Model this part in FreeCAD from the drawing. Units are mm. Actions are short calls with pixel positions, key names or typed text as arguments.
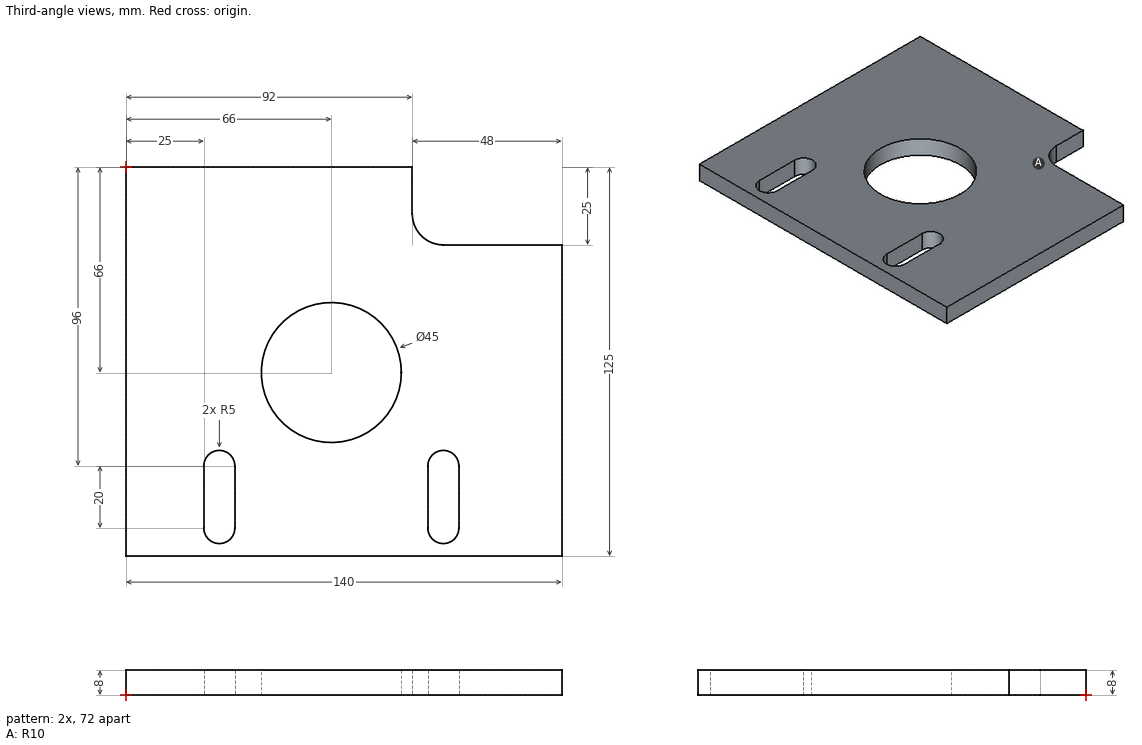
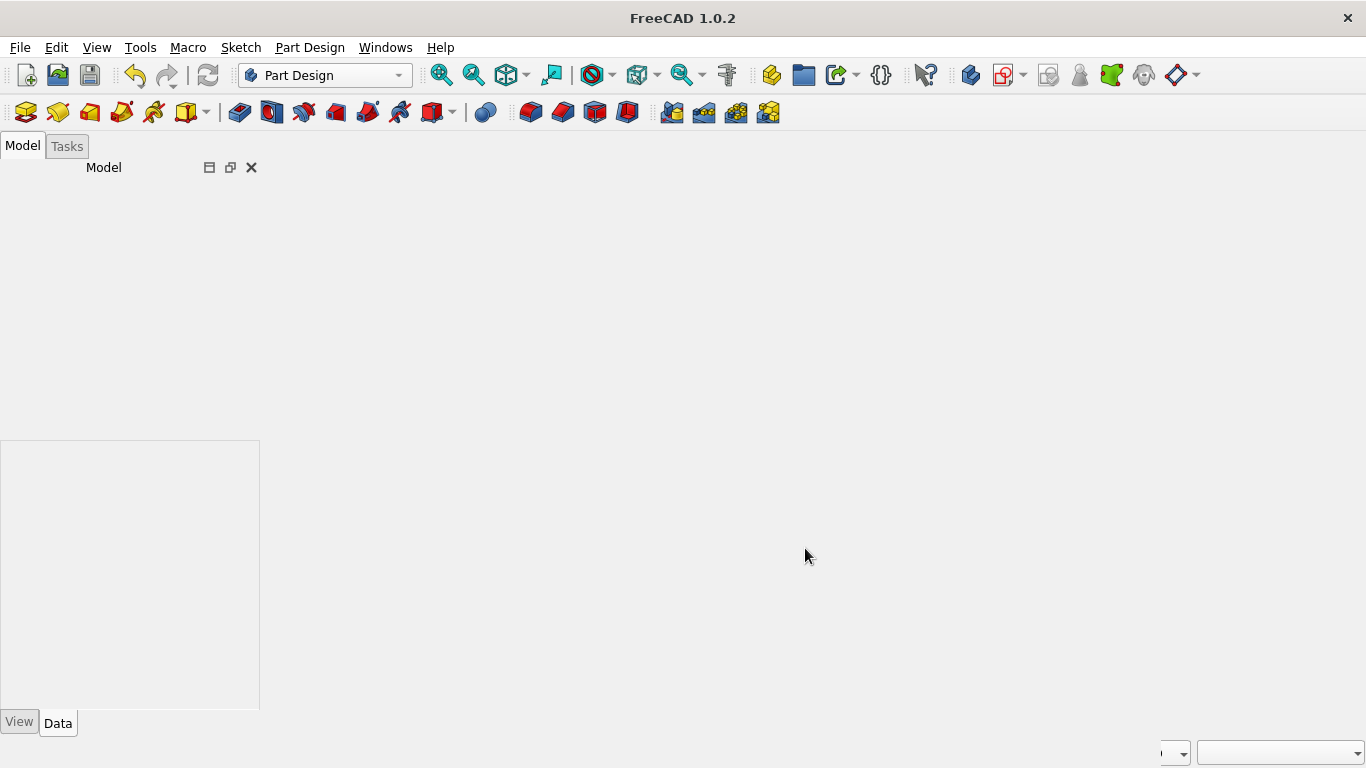
click(26, 76)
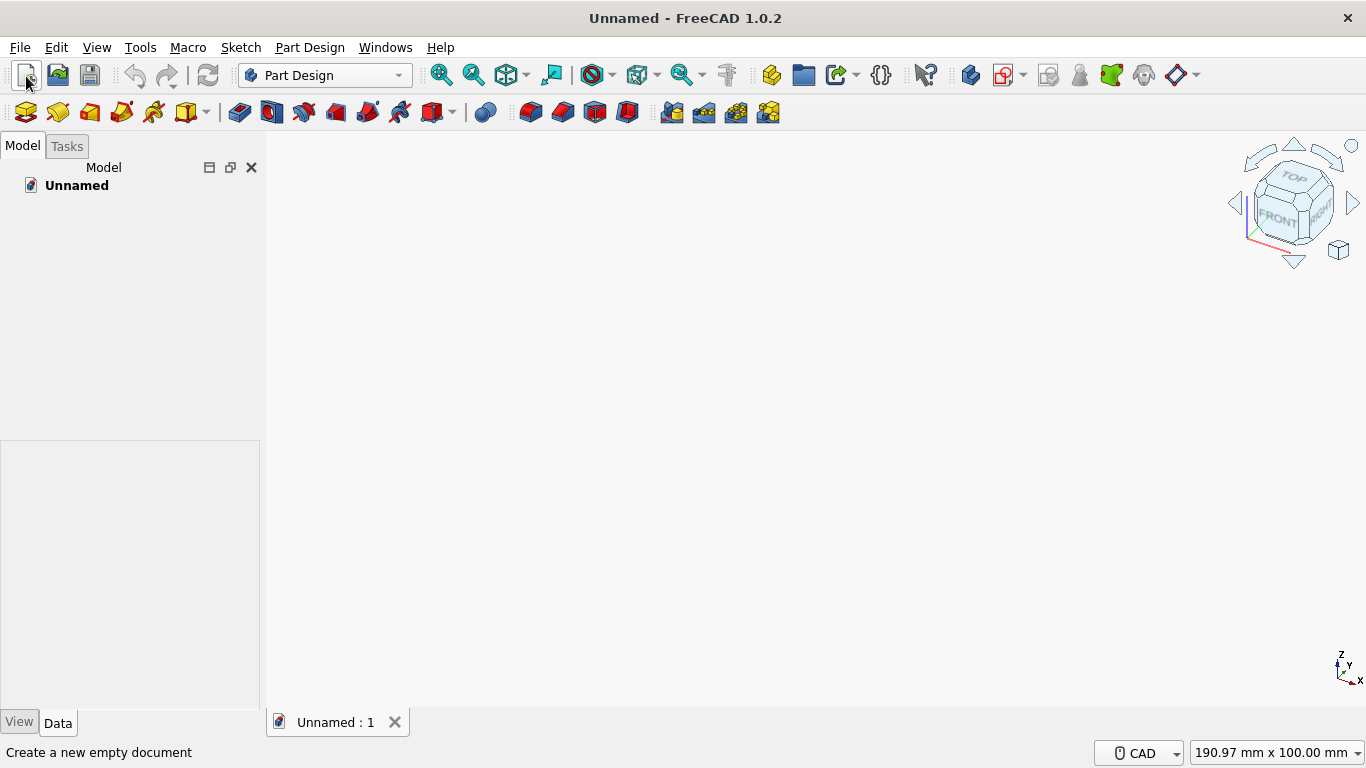
click(1004, 76)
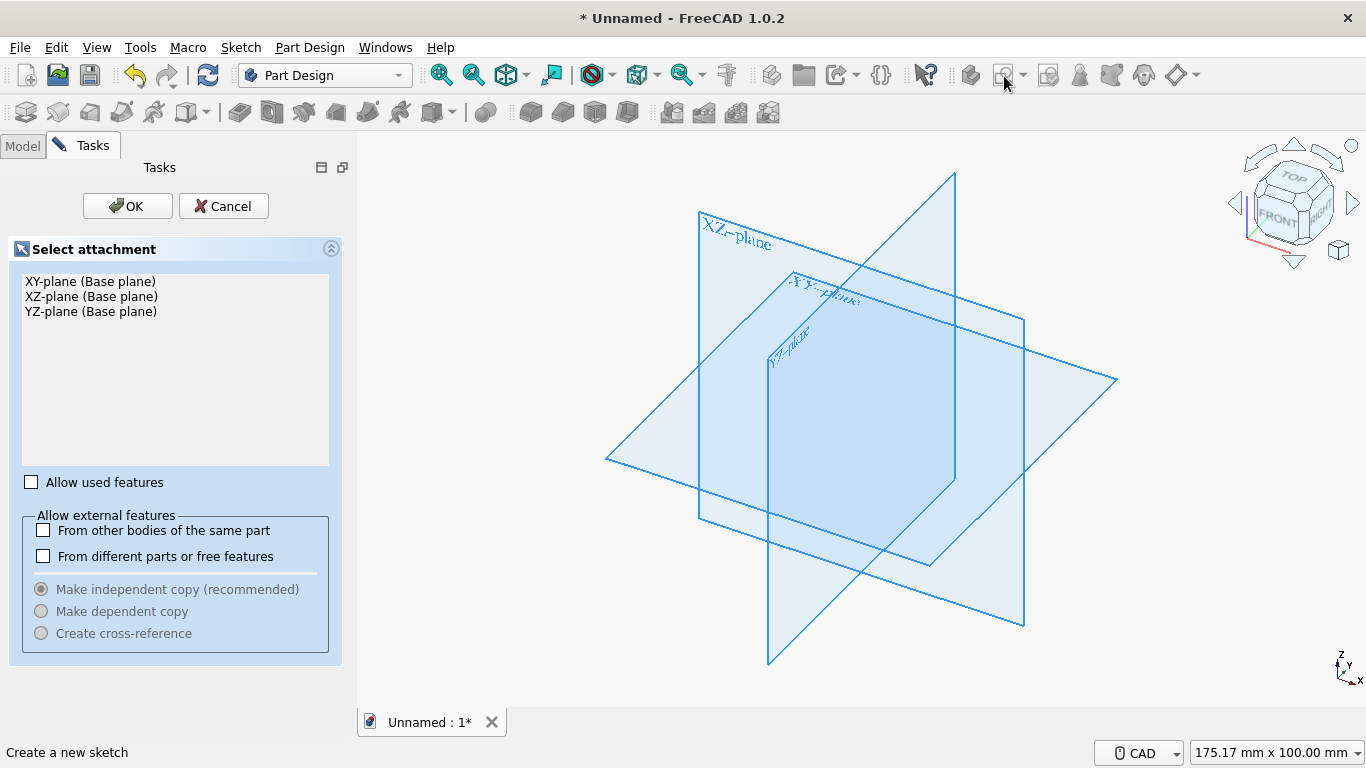
click(82, 282)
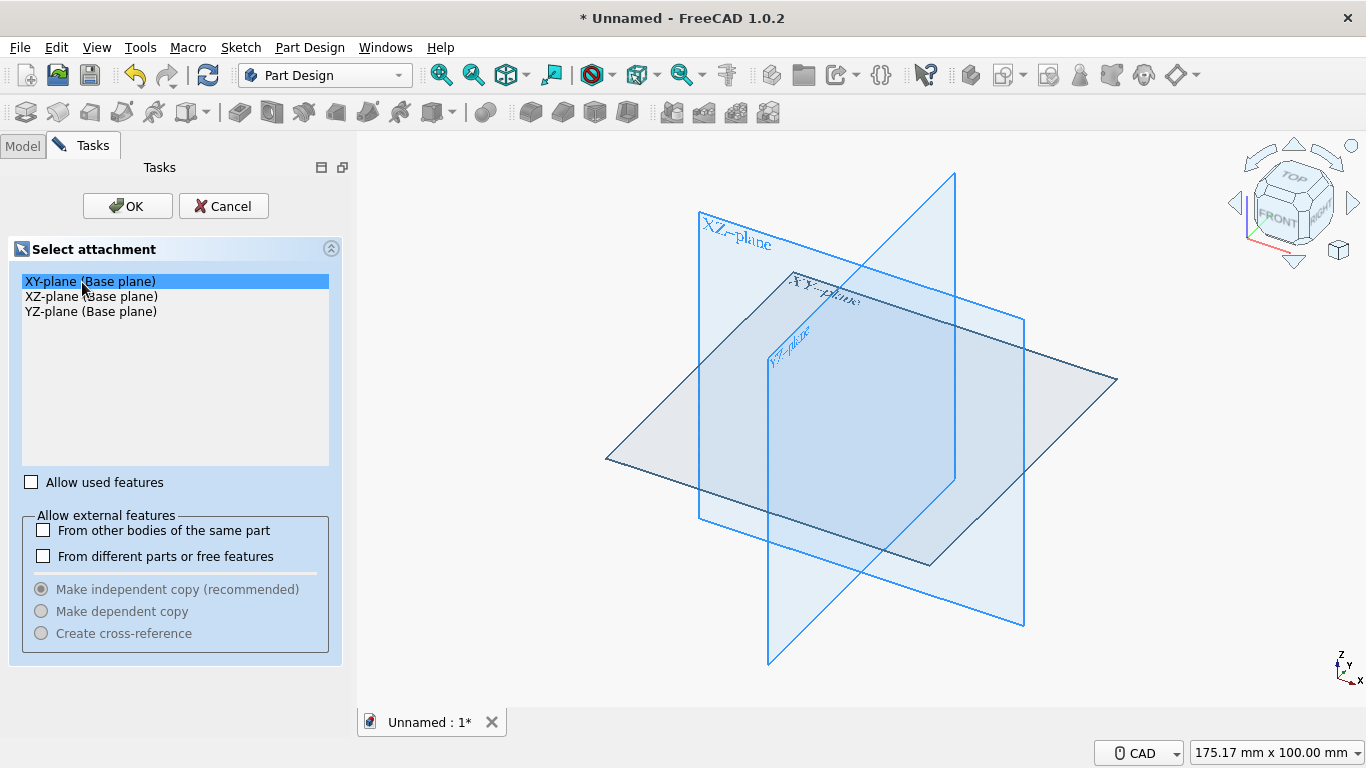
click(128, 206)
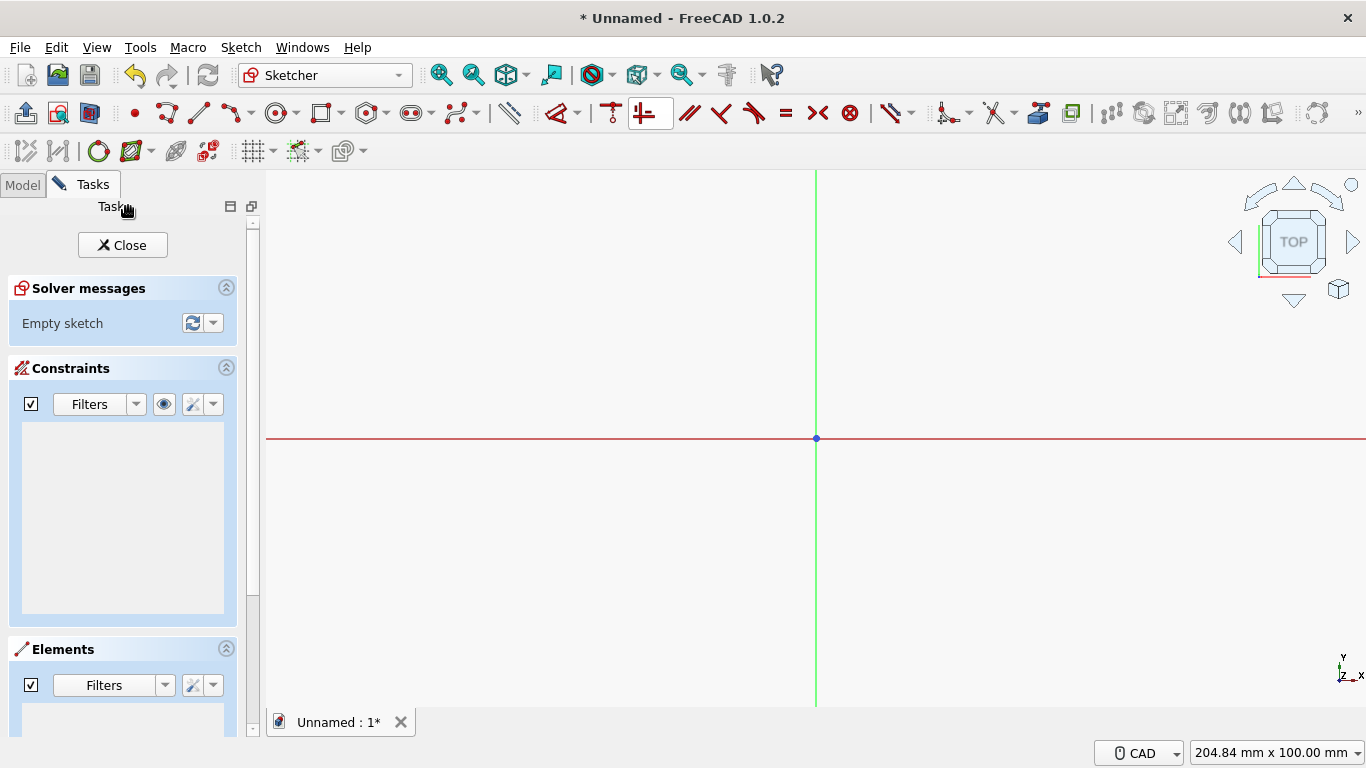
scroll(385, 198, down, 4)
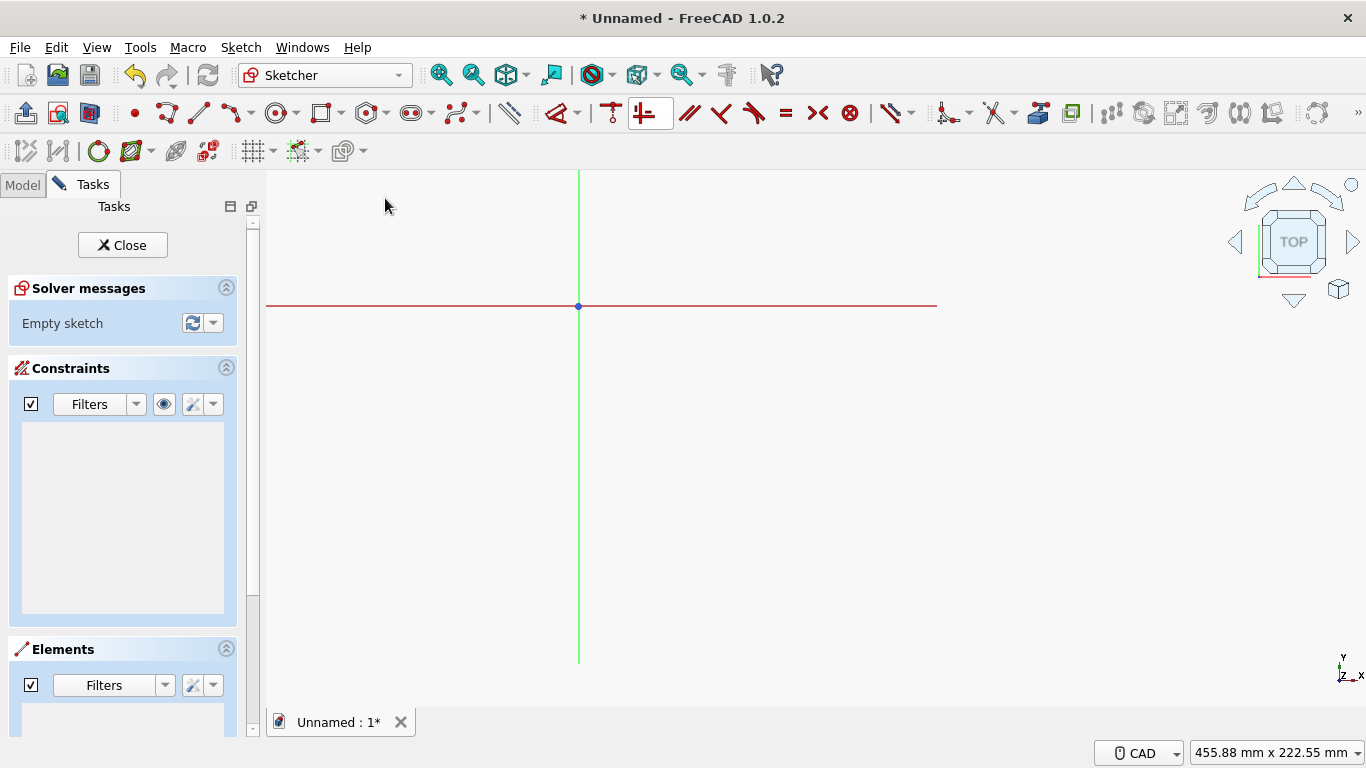
key(g)
key(r)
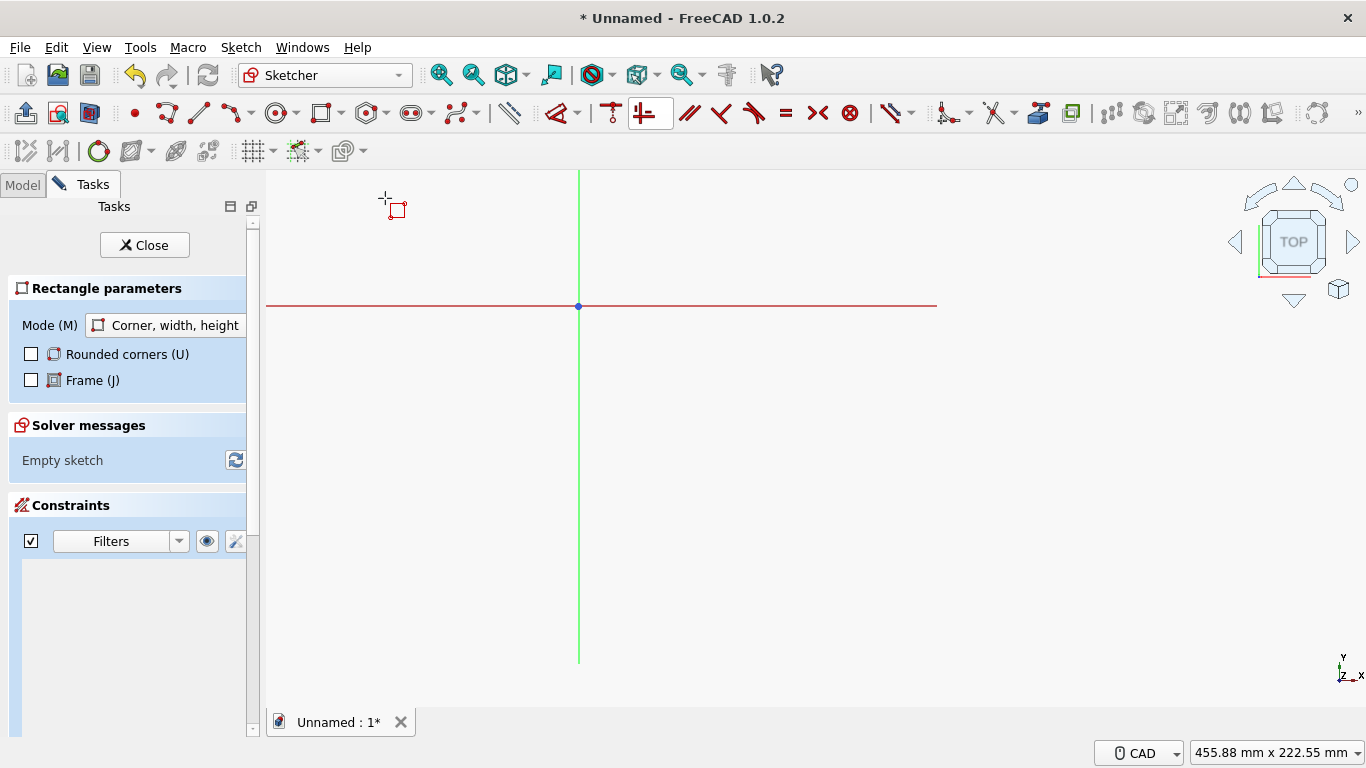
click(579, 306)
move(917, 608)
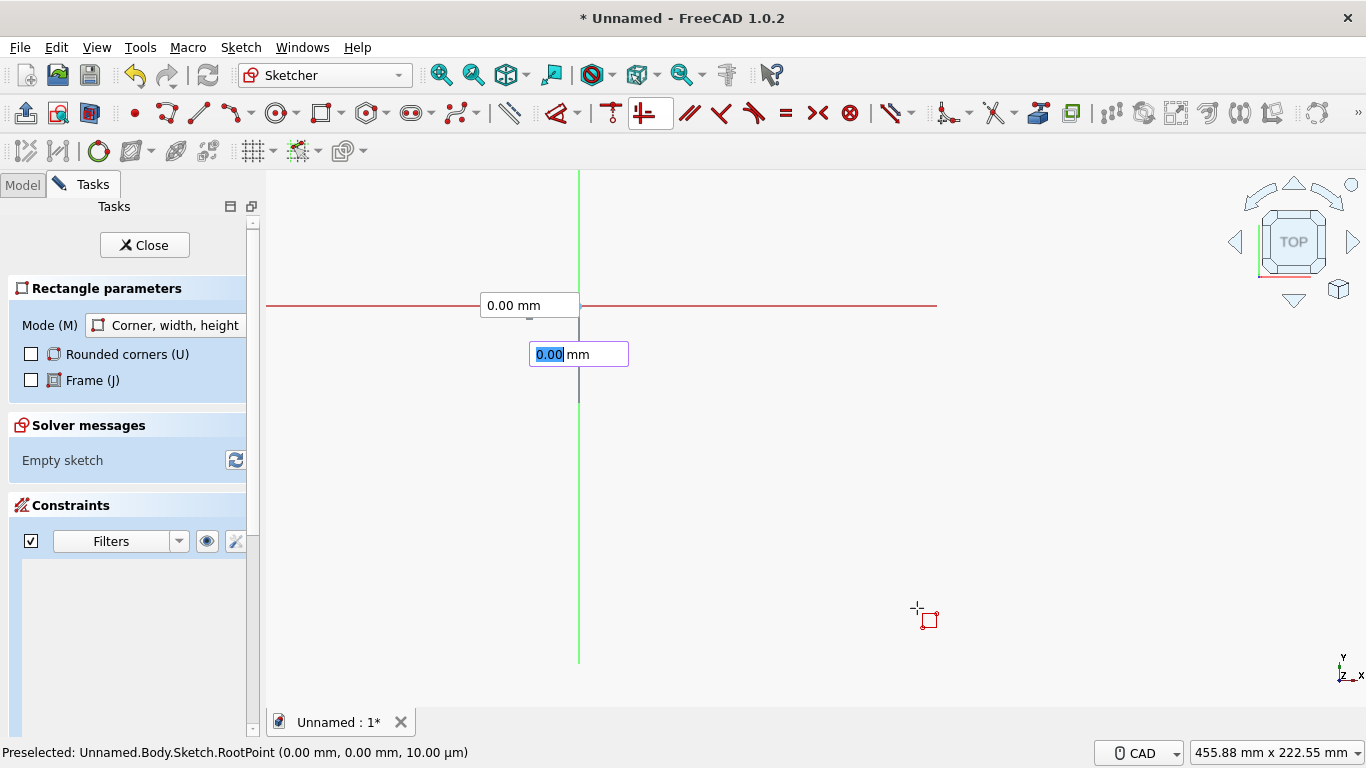
text(140)
key(Tab)
text(125)
key(Return)
key(Escape)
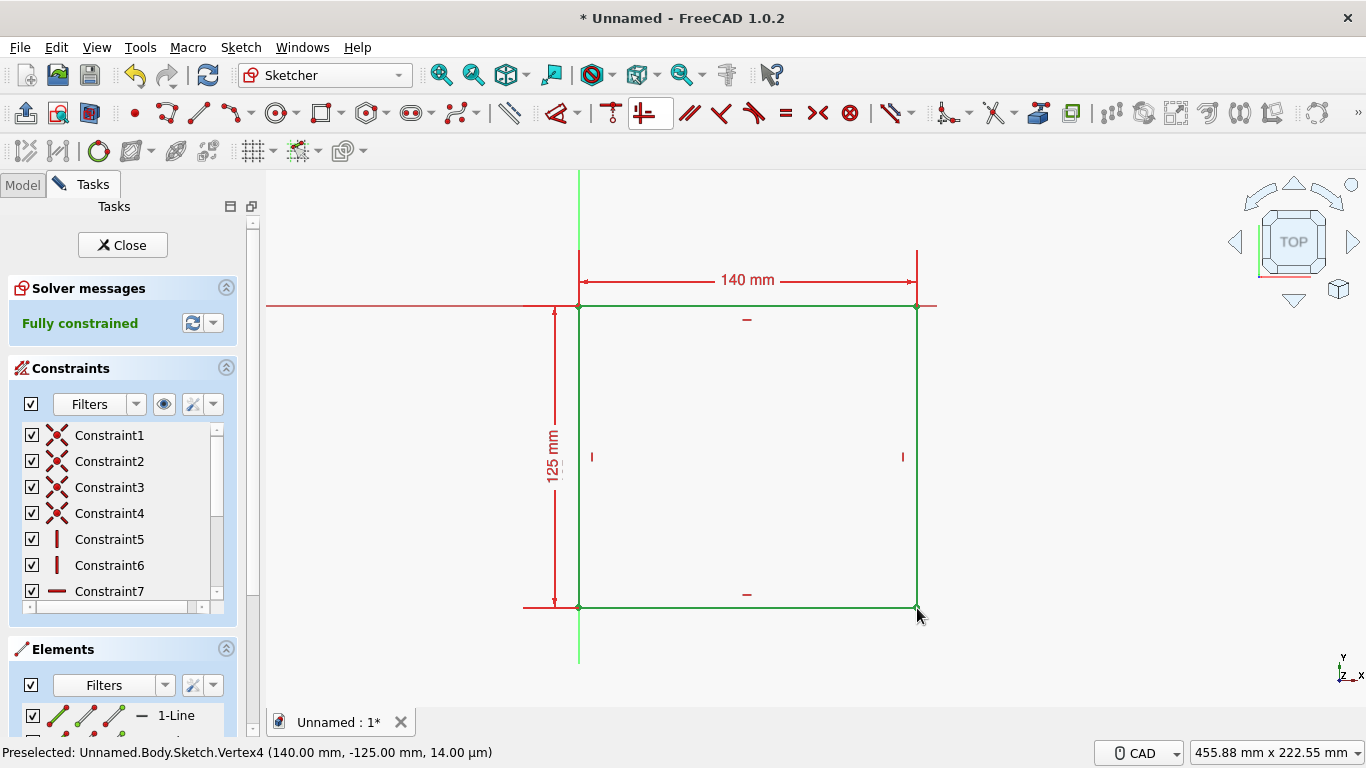
click(123, 245)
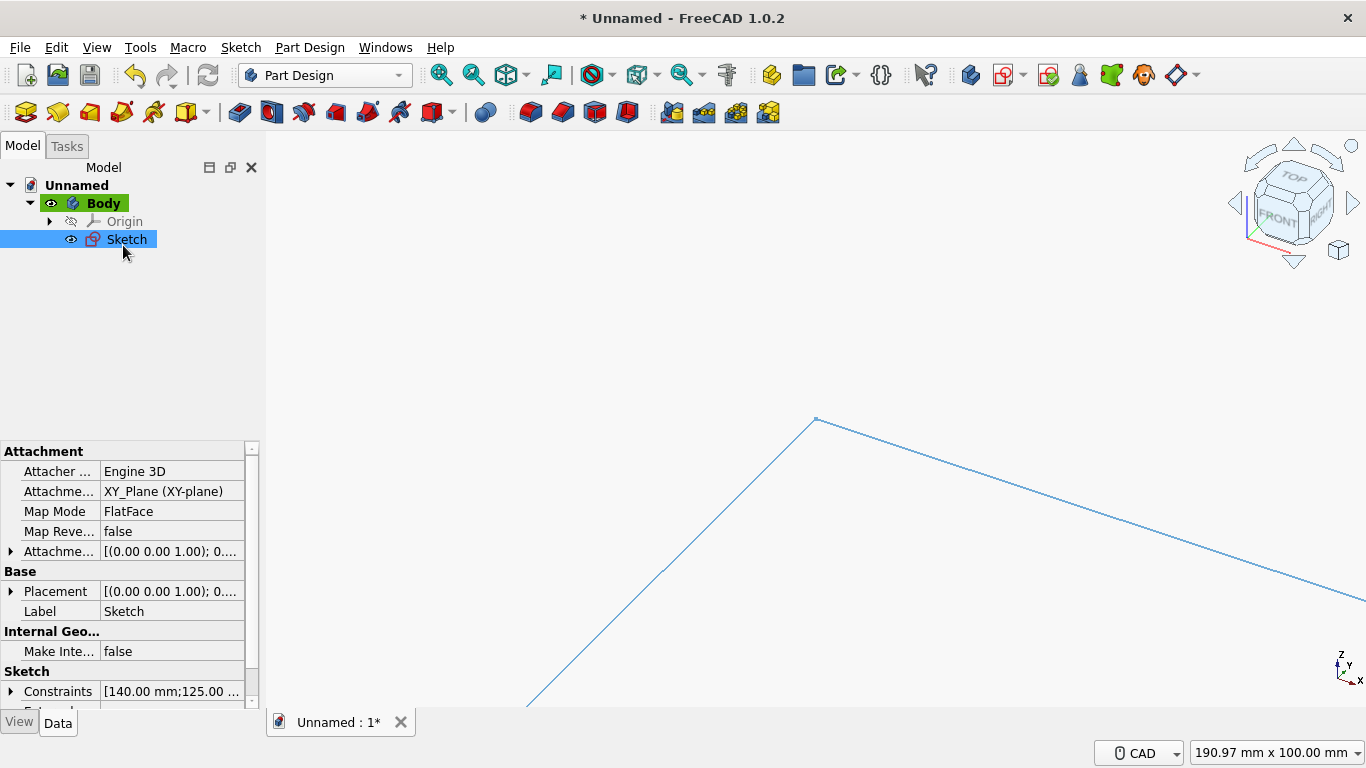
click(26, 112)